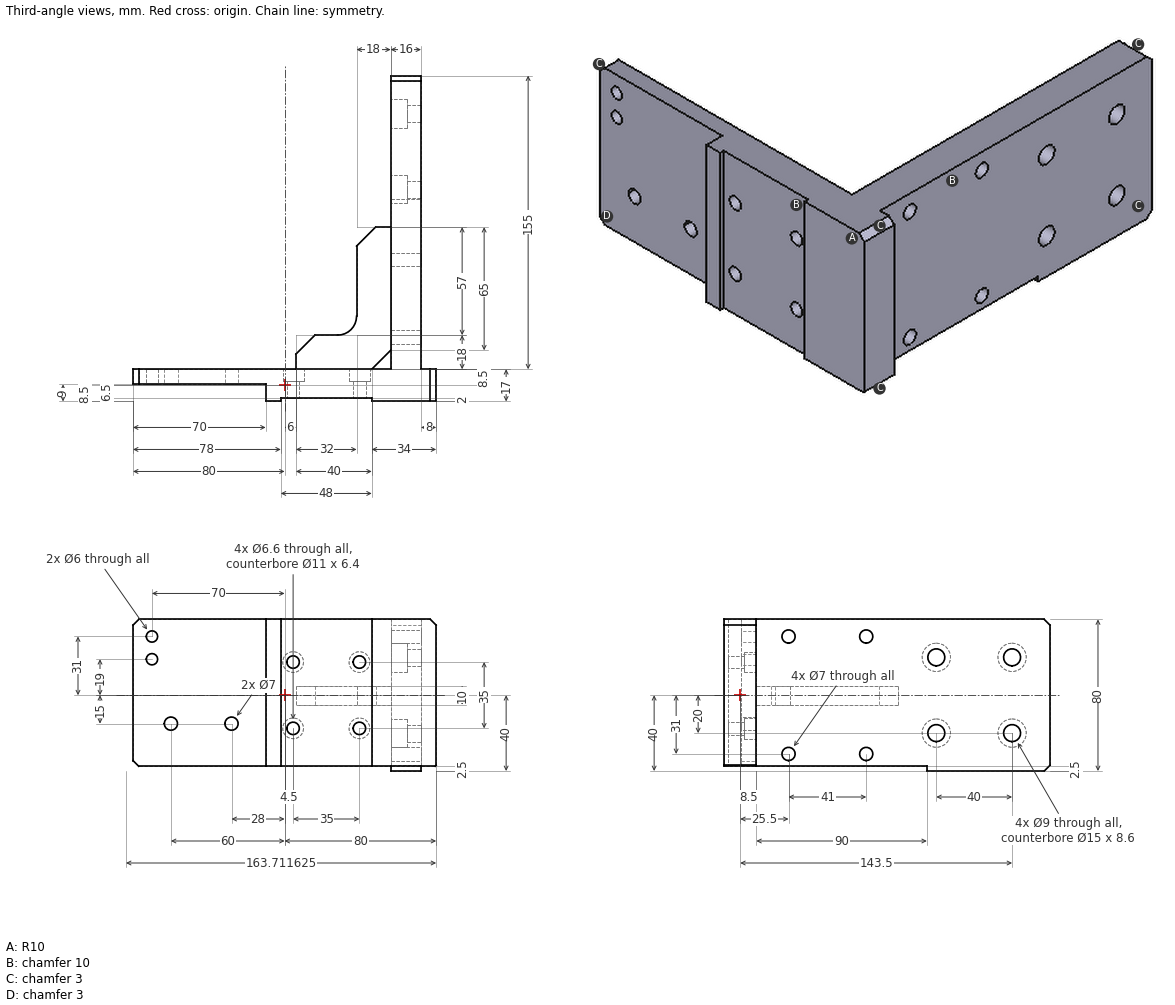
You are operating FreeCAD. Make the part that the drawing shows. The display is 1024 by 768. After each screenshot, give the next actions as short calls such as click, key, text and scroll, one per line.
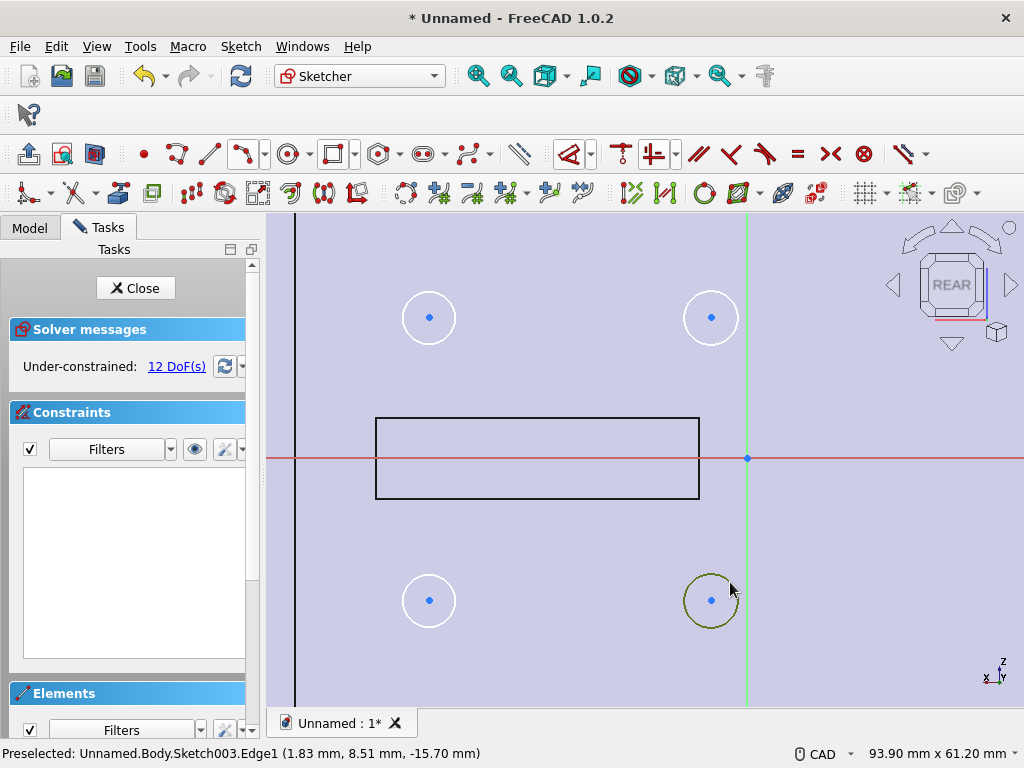
click(447, 582)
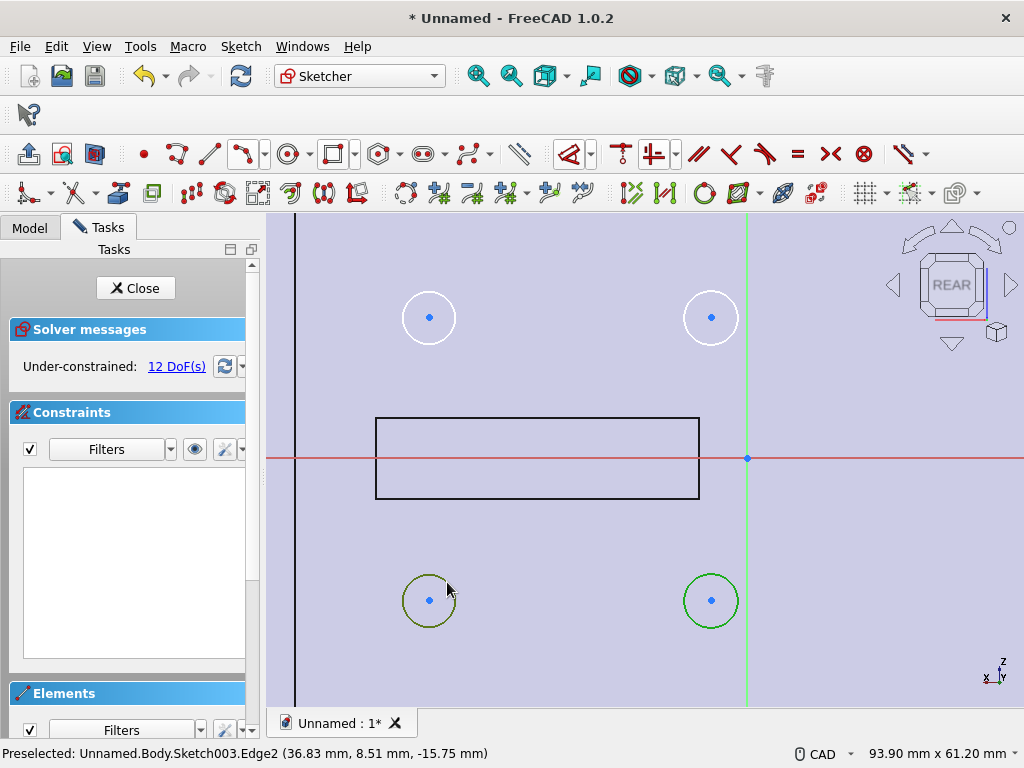
click(447, 299)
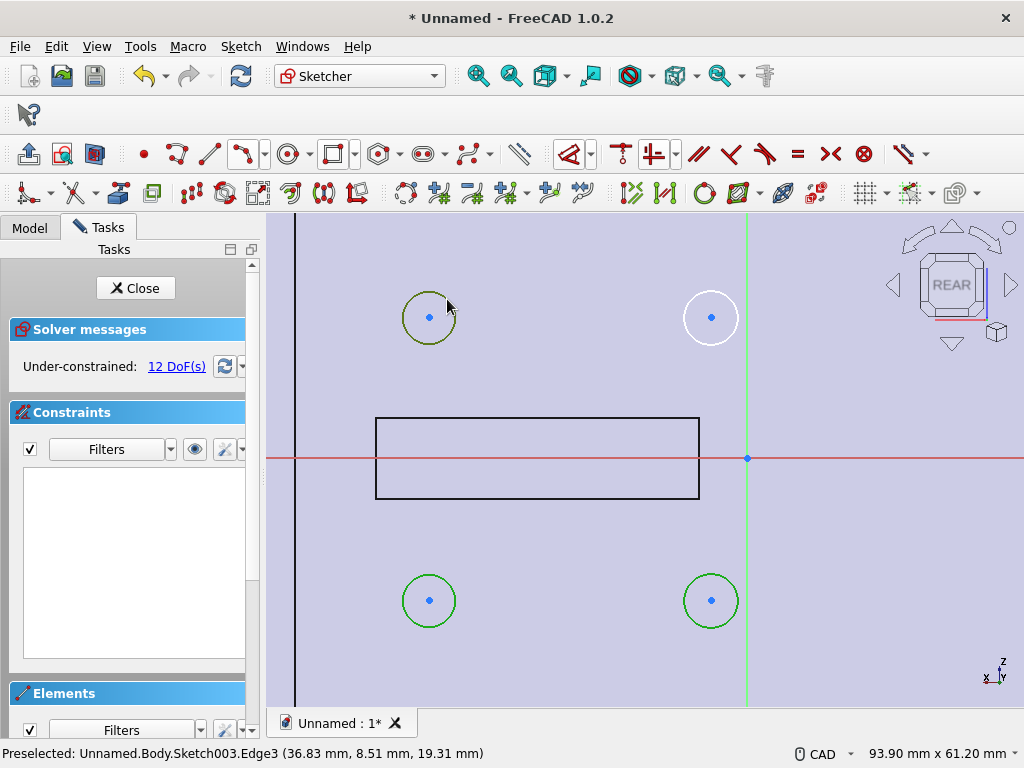
click(730, 299)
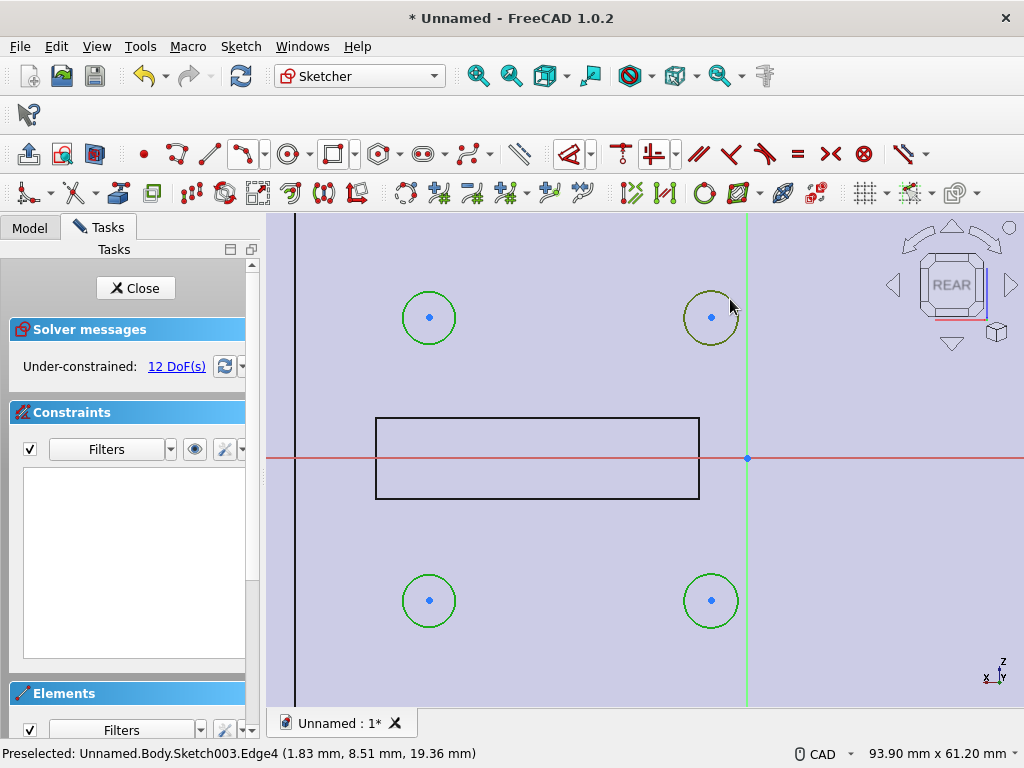
key(e)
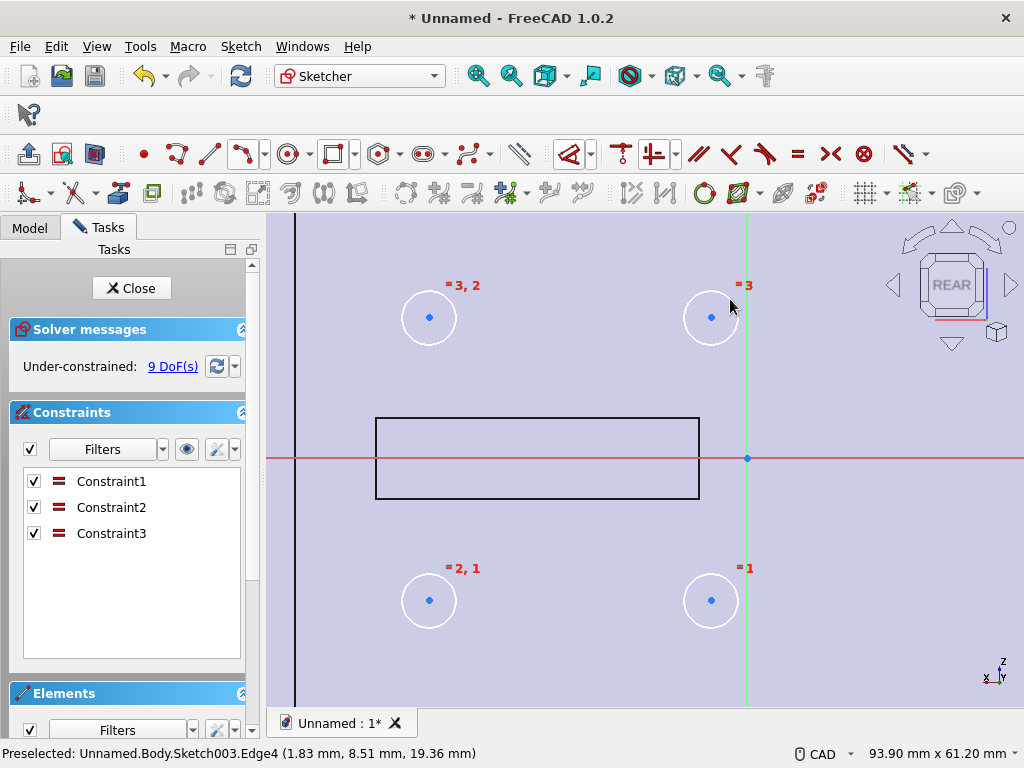
click(429, 601)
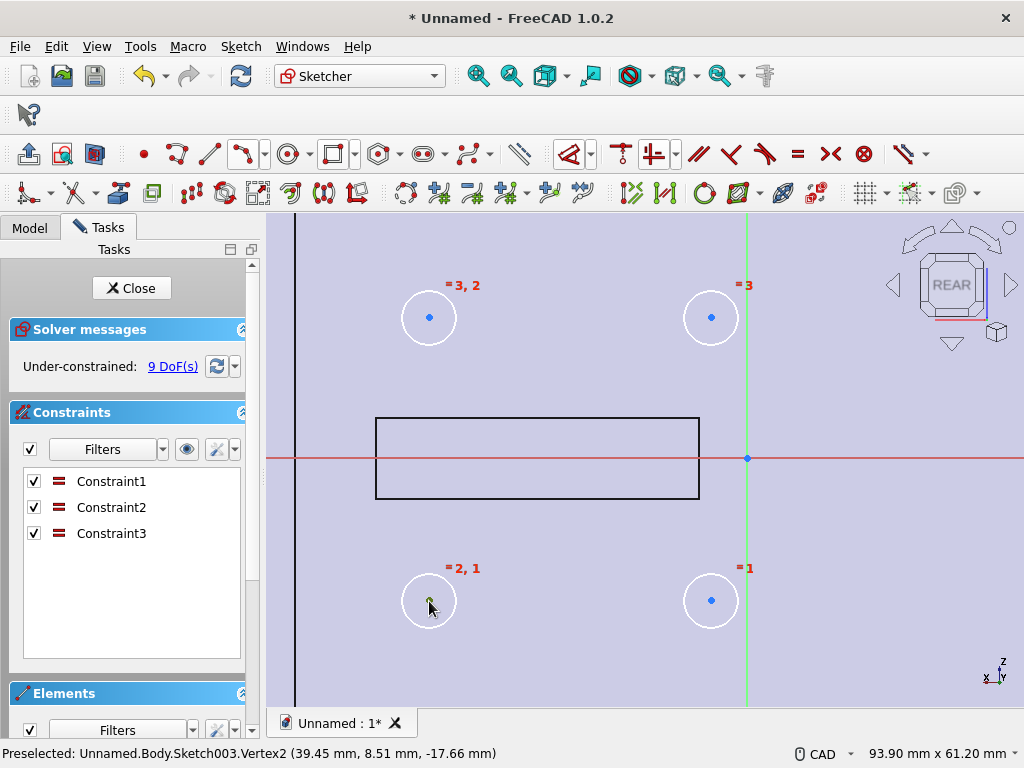
click(429, 318)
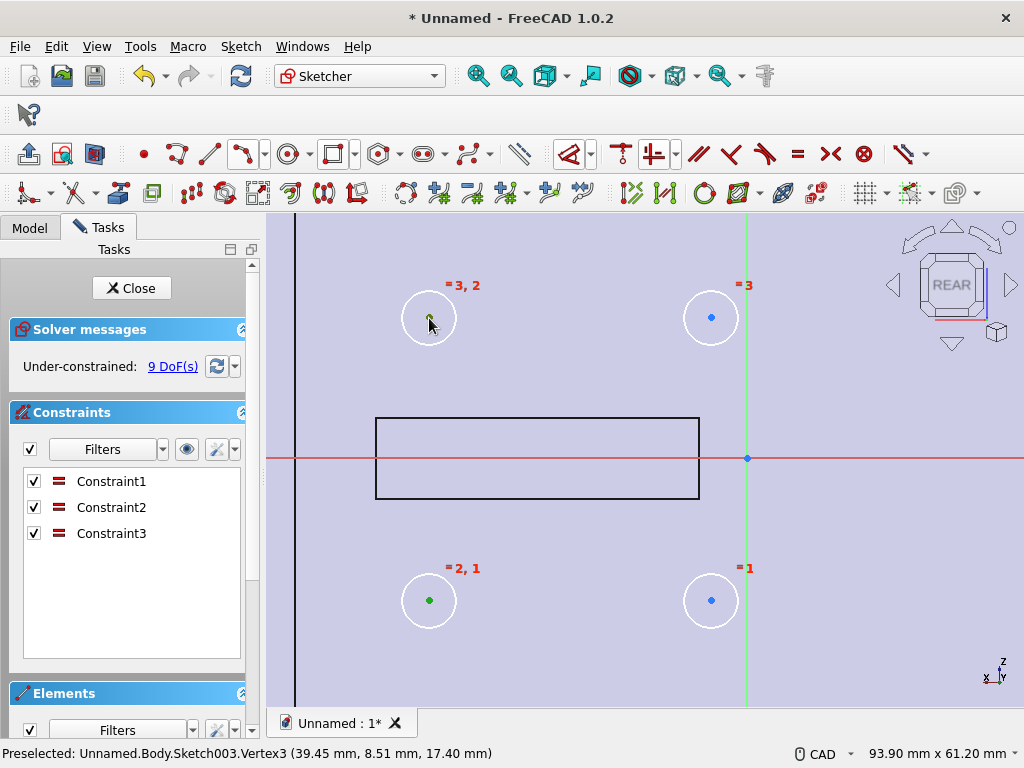
click(334, 458)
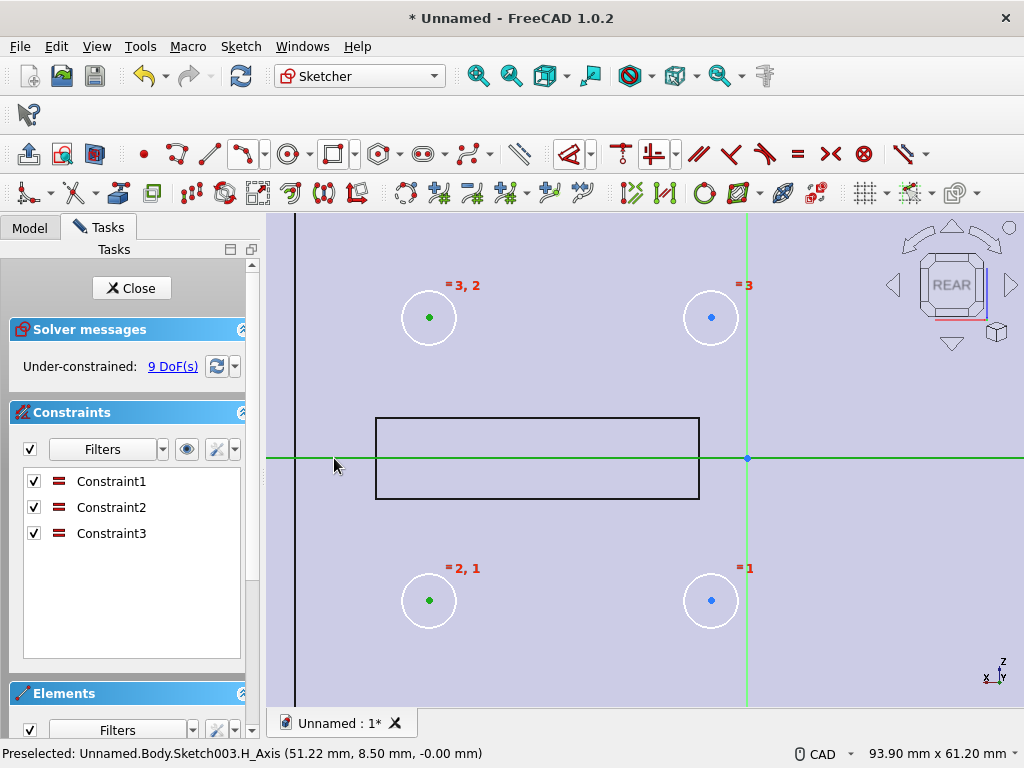
click(831, 154)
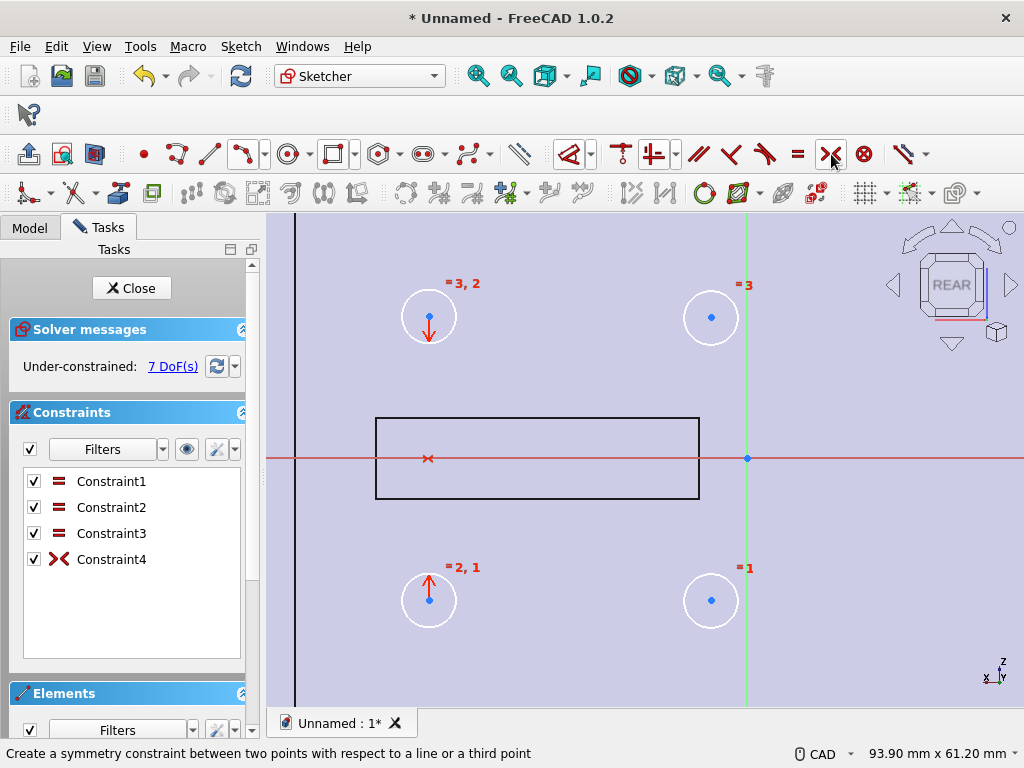
click(711, 601)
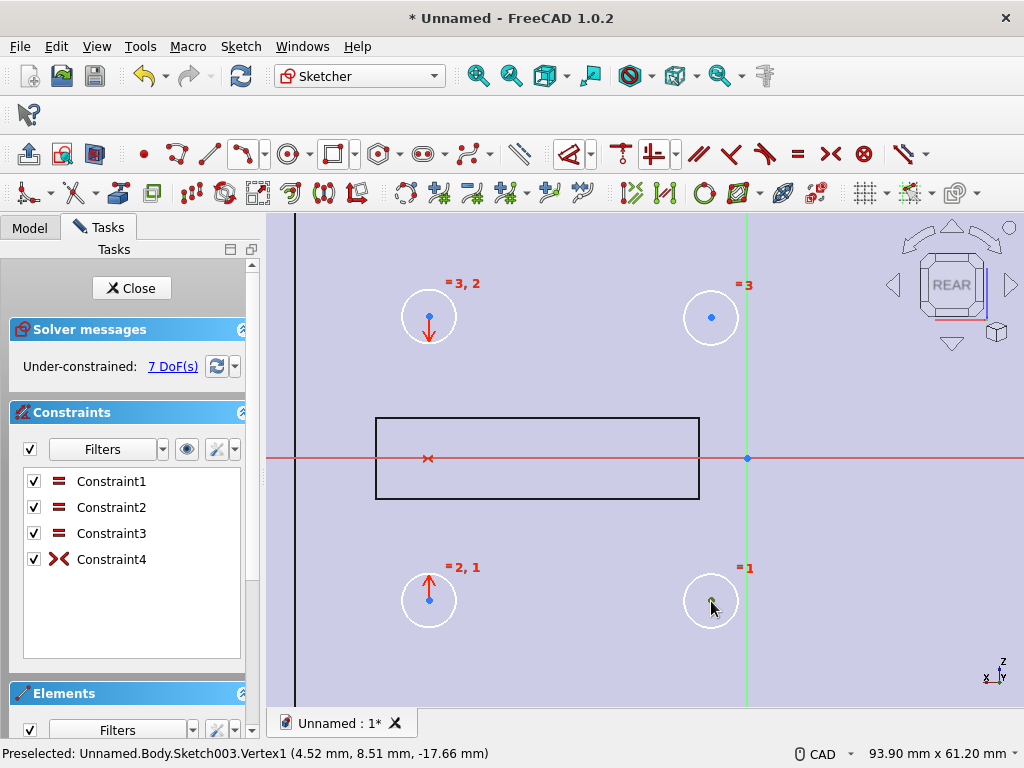
click(711, 318)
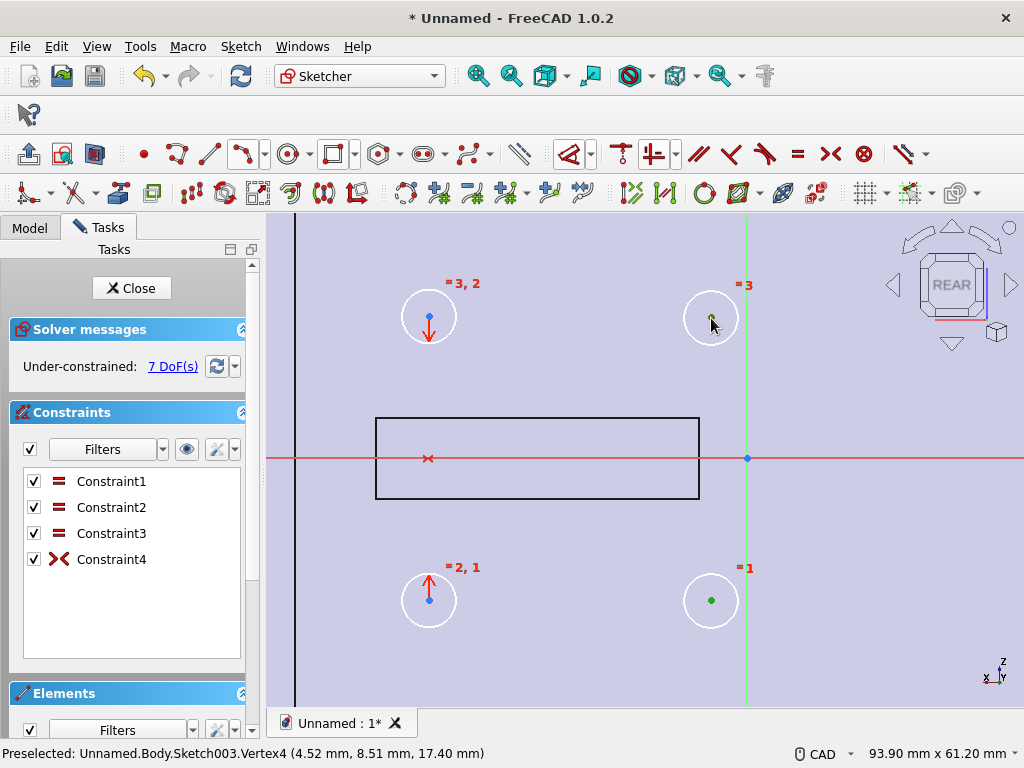
click(334, 458)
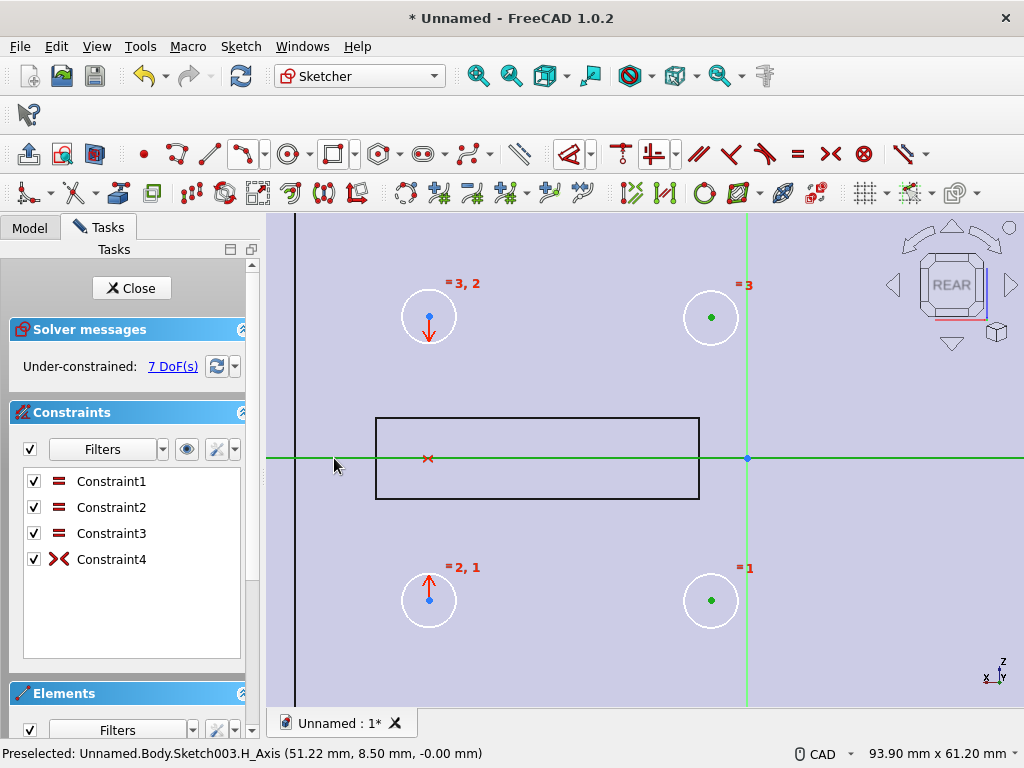
click(831, 154)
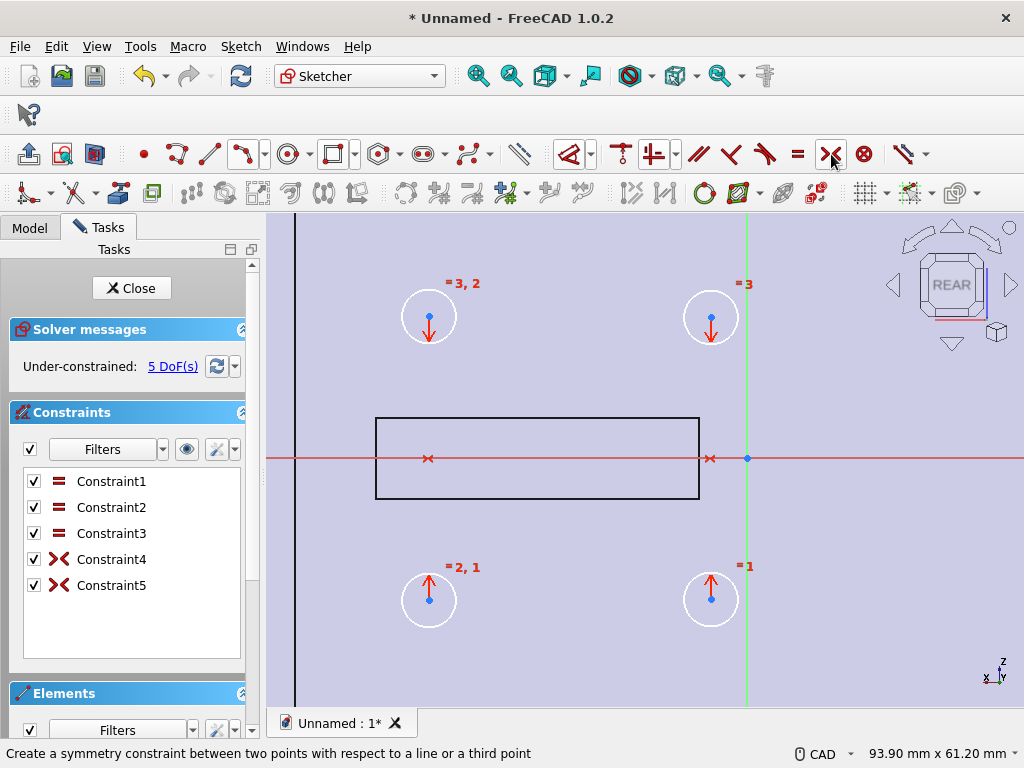
click(730, 580)